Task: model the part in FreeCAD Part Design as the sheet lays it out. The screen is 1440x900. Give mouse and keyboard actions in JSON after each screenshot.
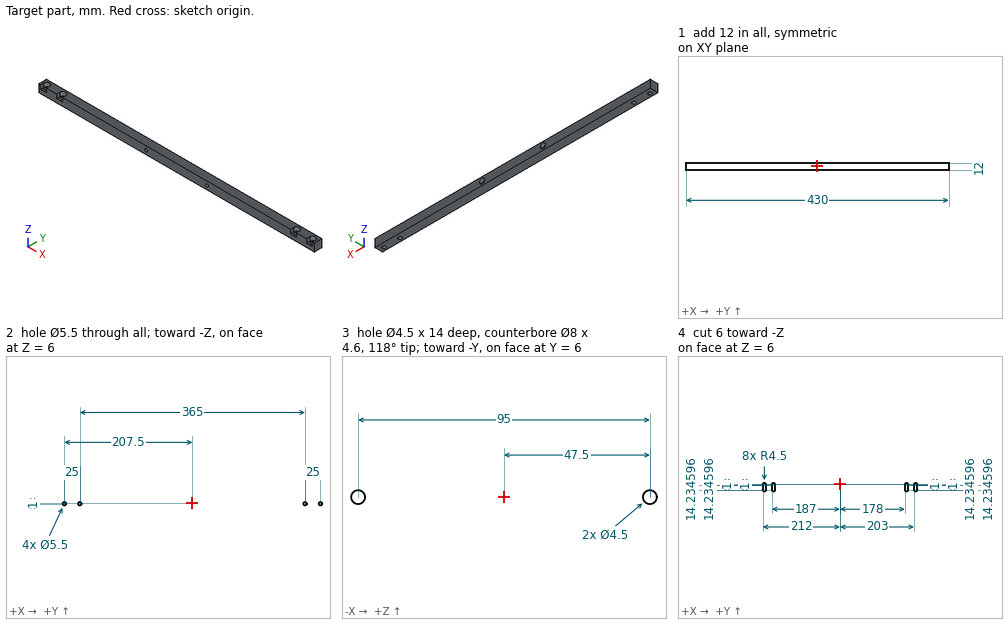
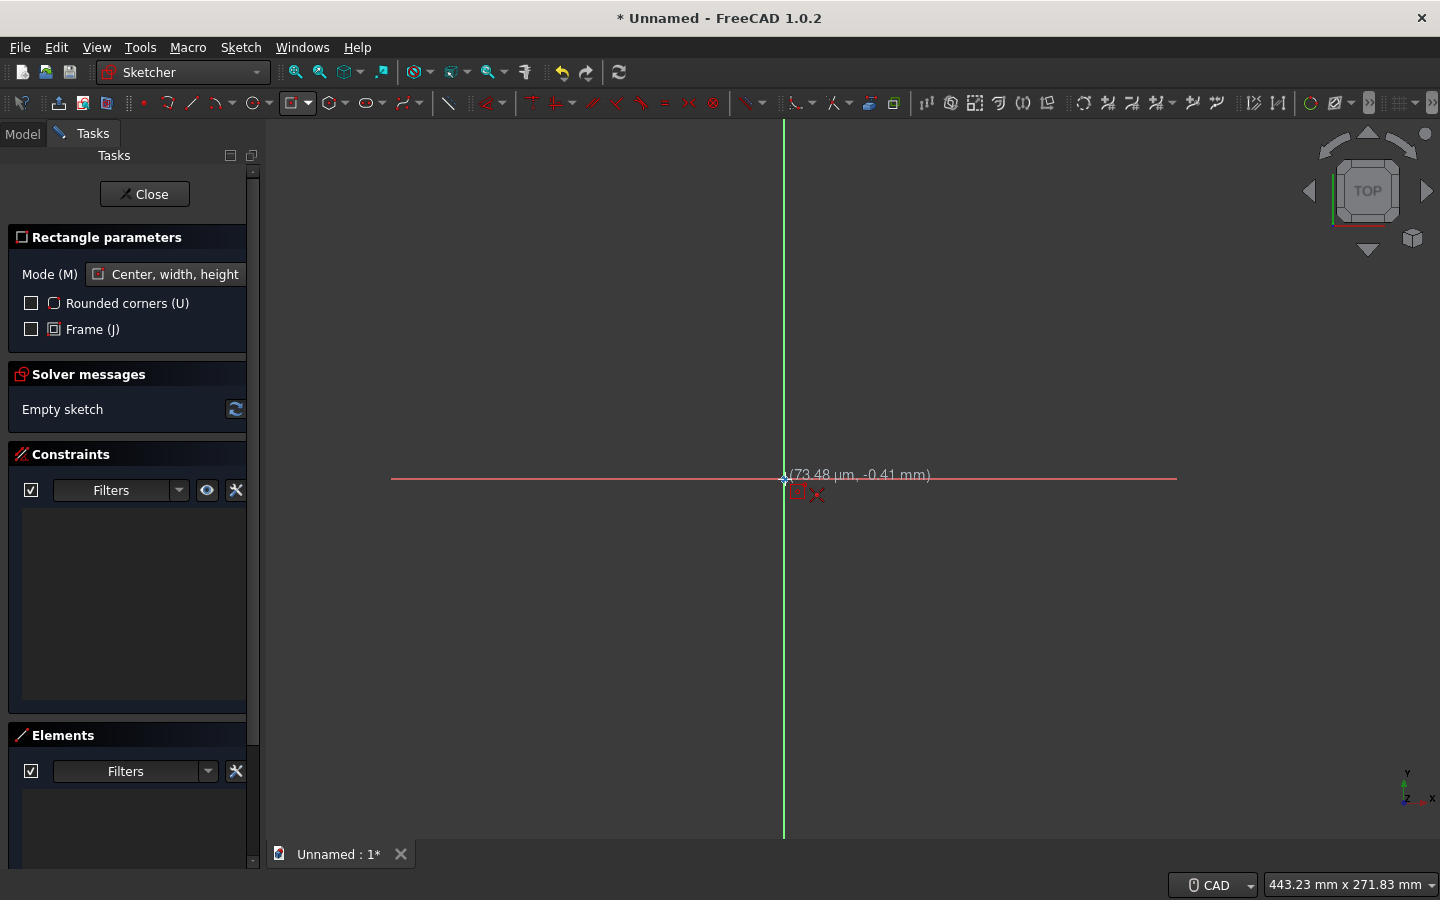
{"action": "left_click", "coordinate": [784, 479]}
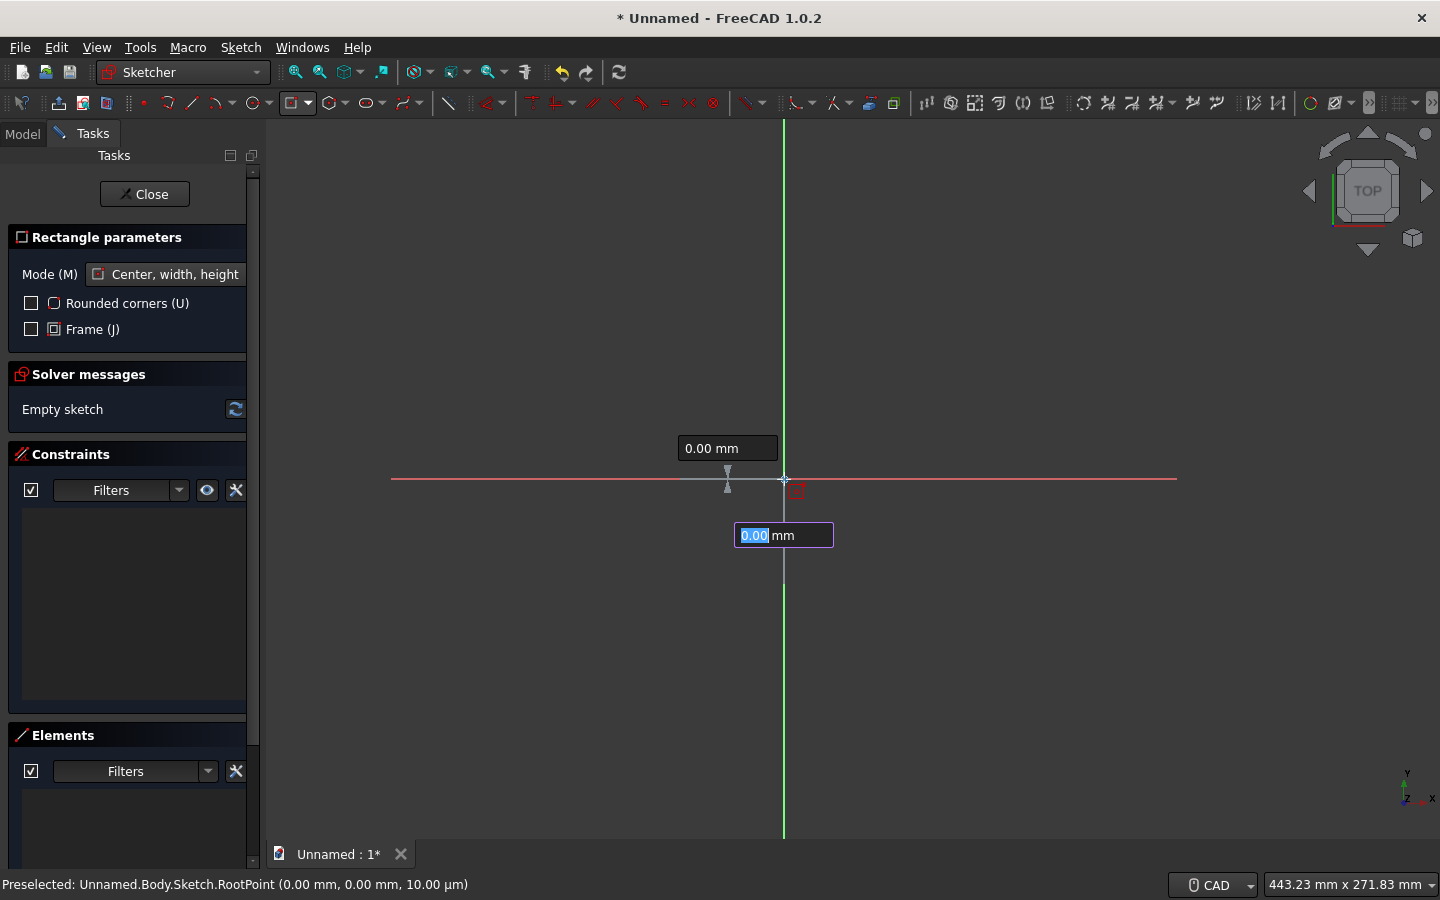
{"action": "scroll", "coordinate": [785, 478], "scroll_direction": "down", "scroll_amount": 2}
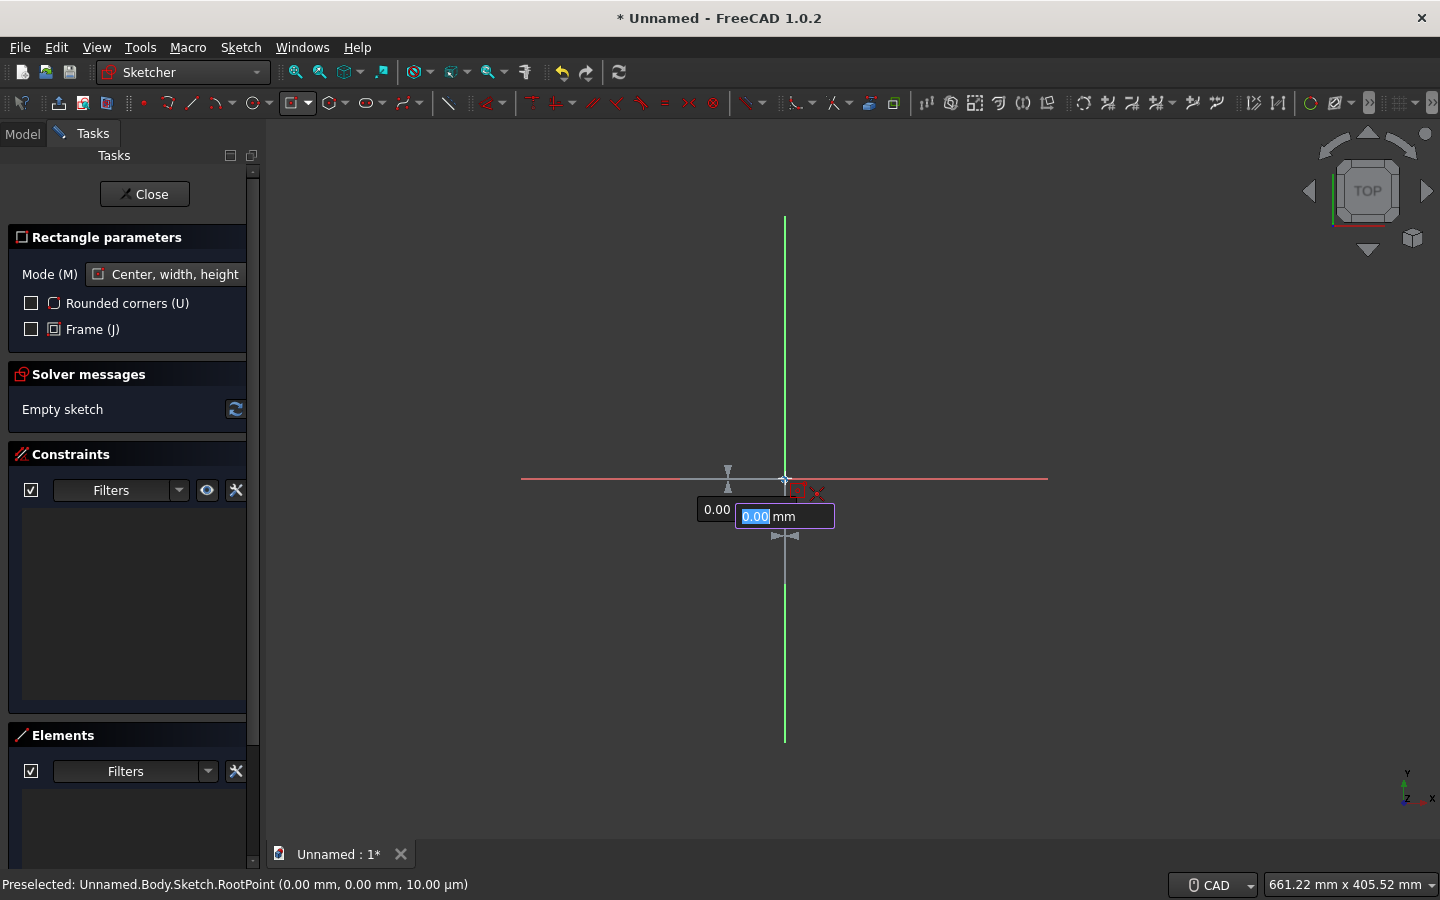
{"action": "scroll", "coordinate": [1167, 468], "scroll_direction": "up", "scroll_amount": 2}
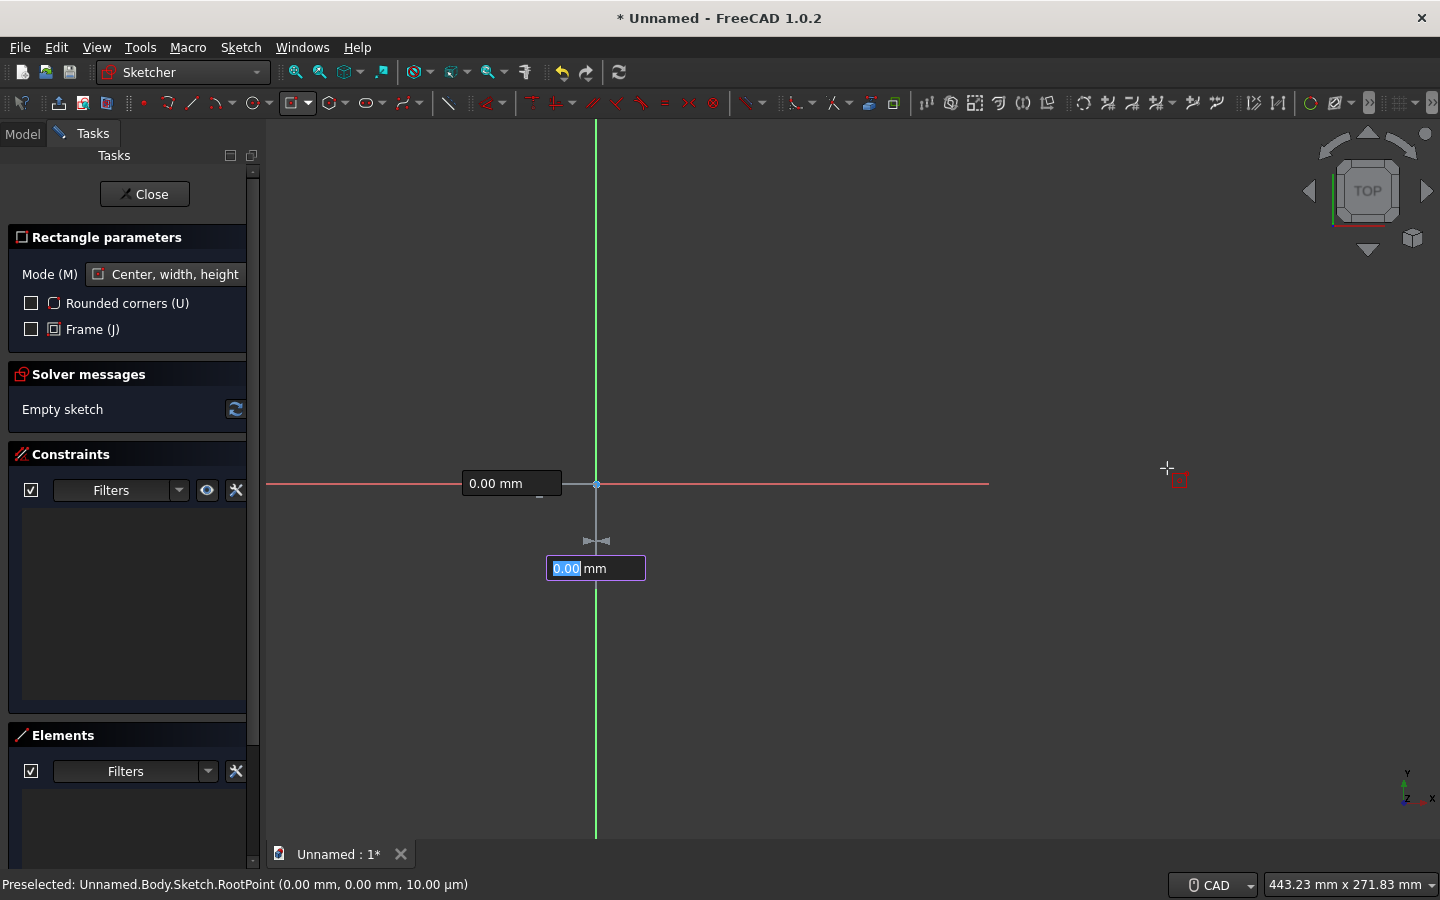
{"action": "left_click", "coordinate": [1166, 468]}
{"action": "key", "text": "Escape"}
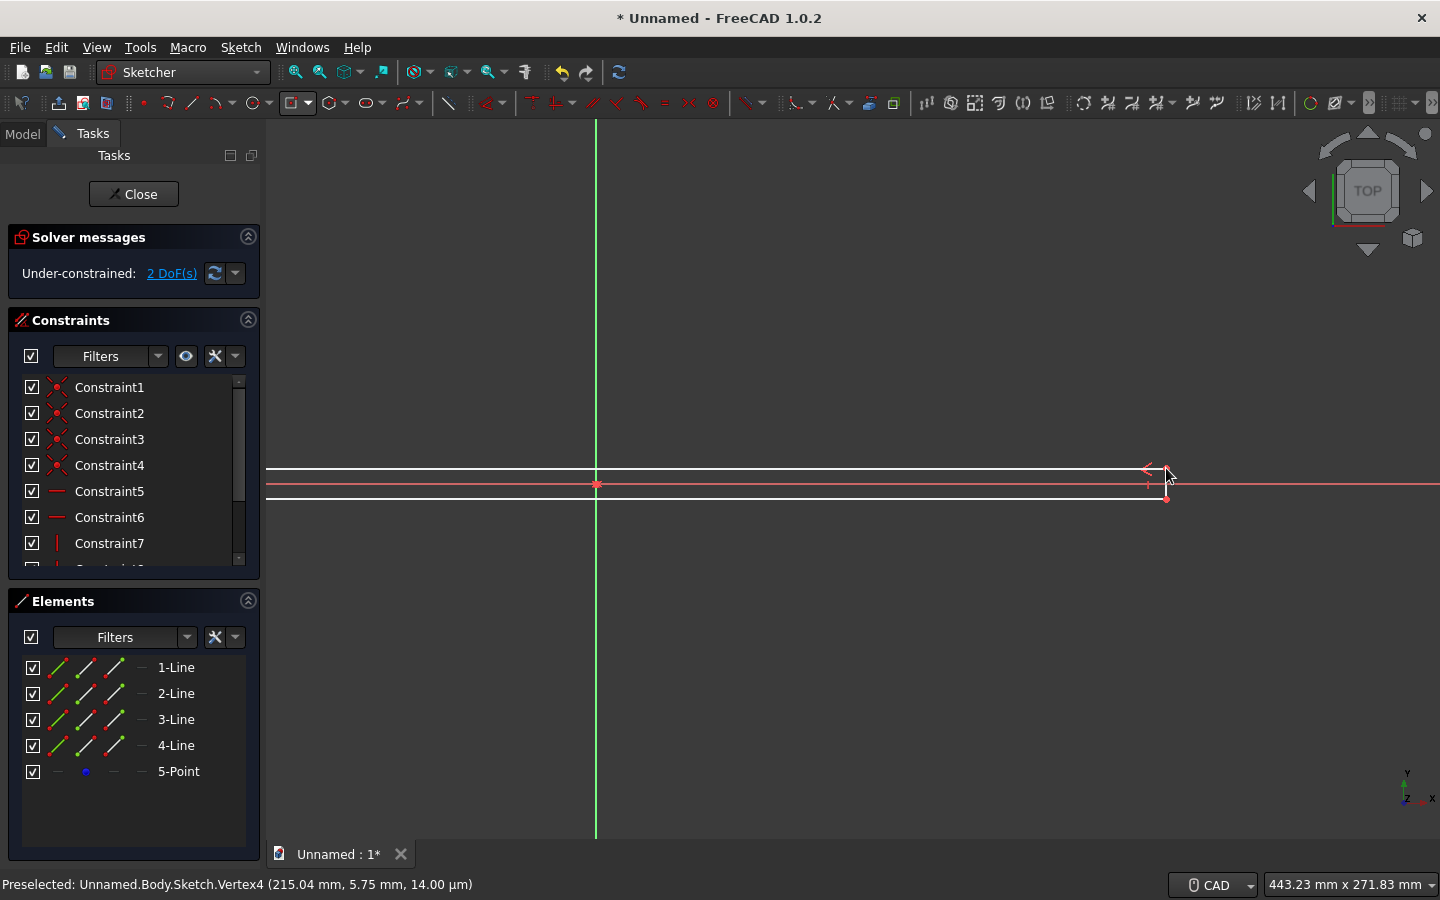
{"action": "left_click", "coordinate": [486, 104]}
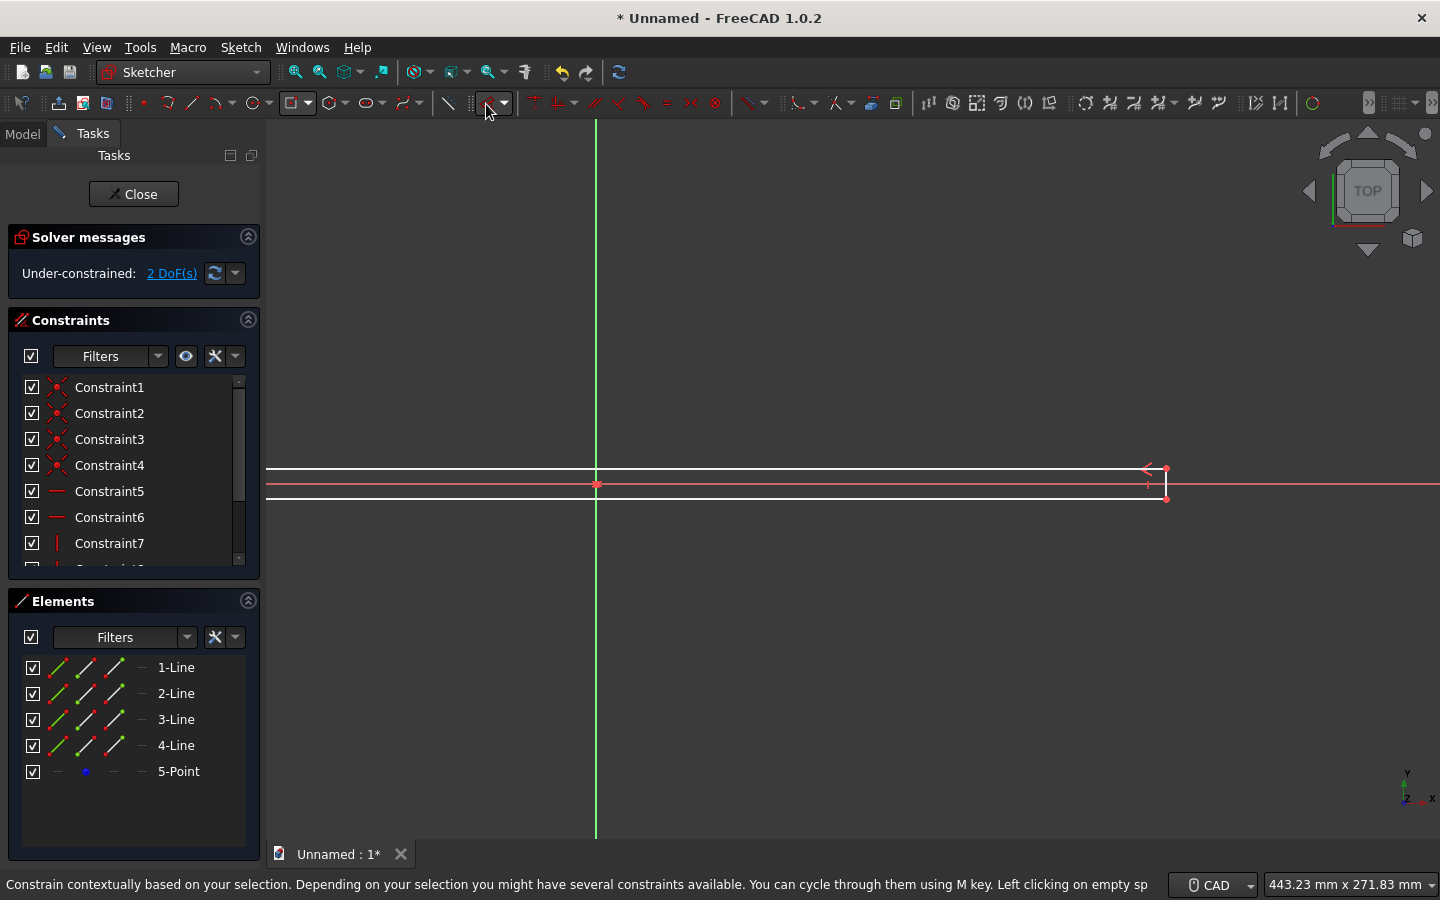
{"action": "scroll", "coordinate": [1166, 487], "scroll_direction": "up", "scroll_amount": 2}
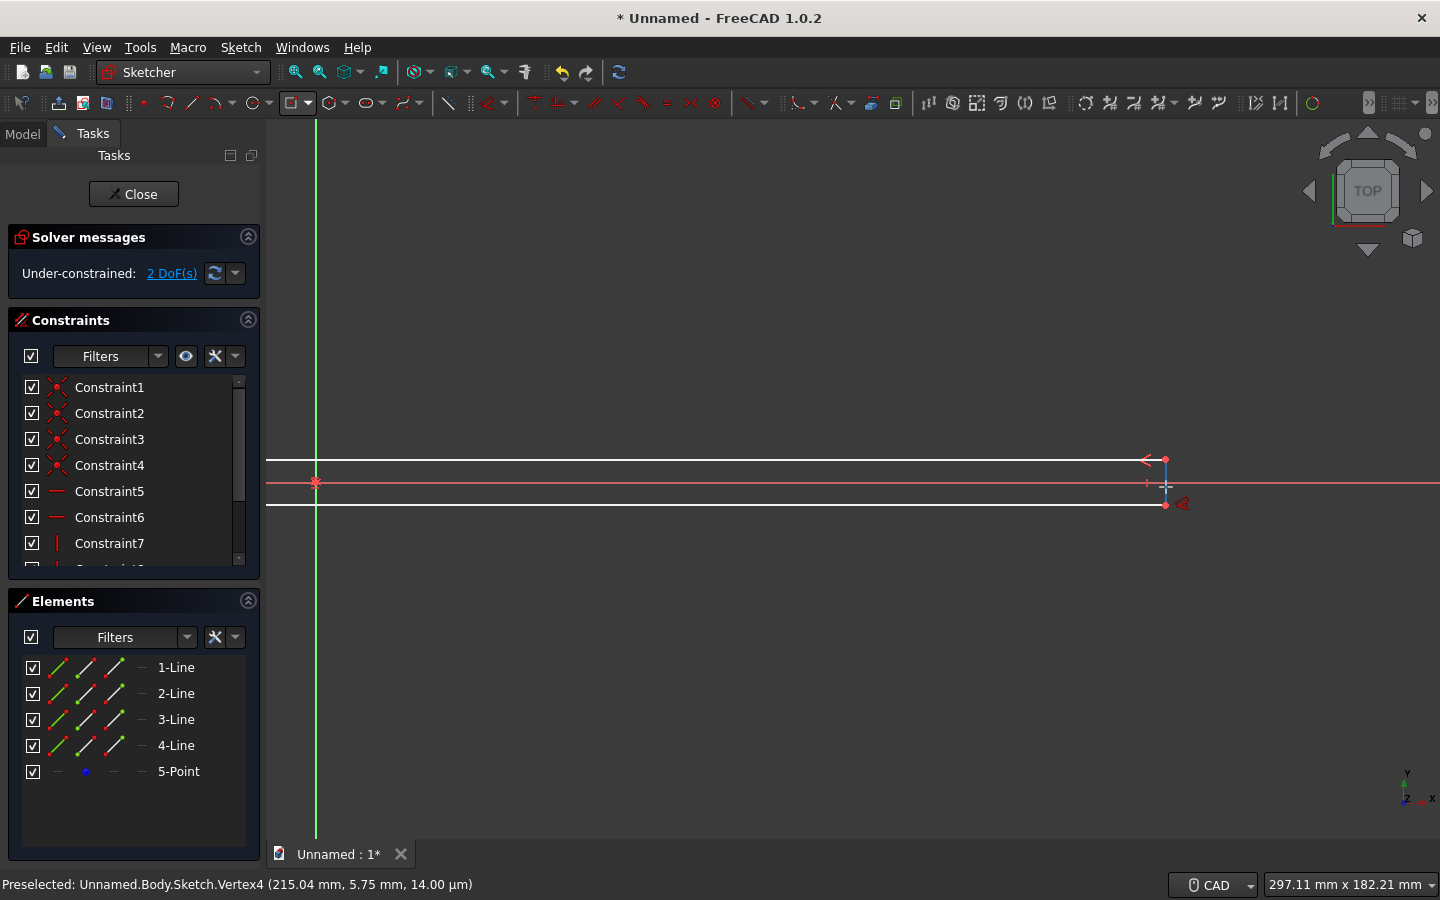
{"action": "left_click", "coordinate": [1166, 487]}
{"action": "left_click", "coordinate": [1200, 467]}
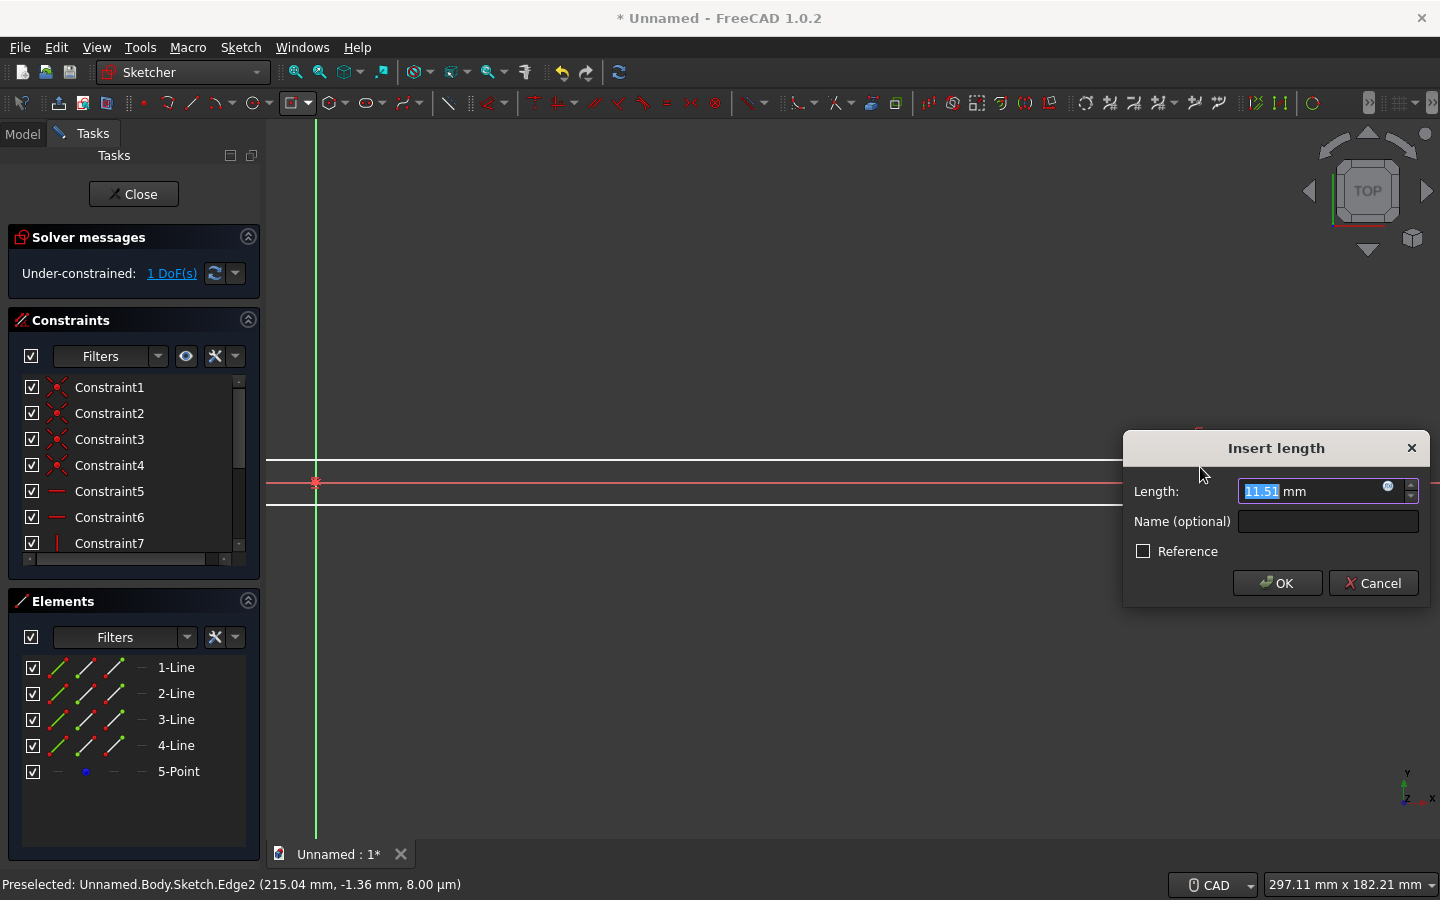
{"action": "type", "text": "12"}
{"action": "key", "text": "Return"}